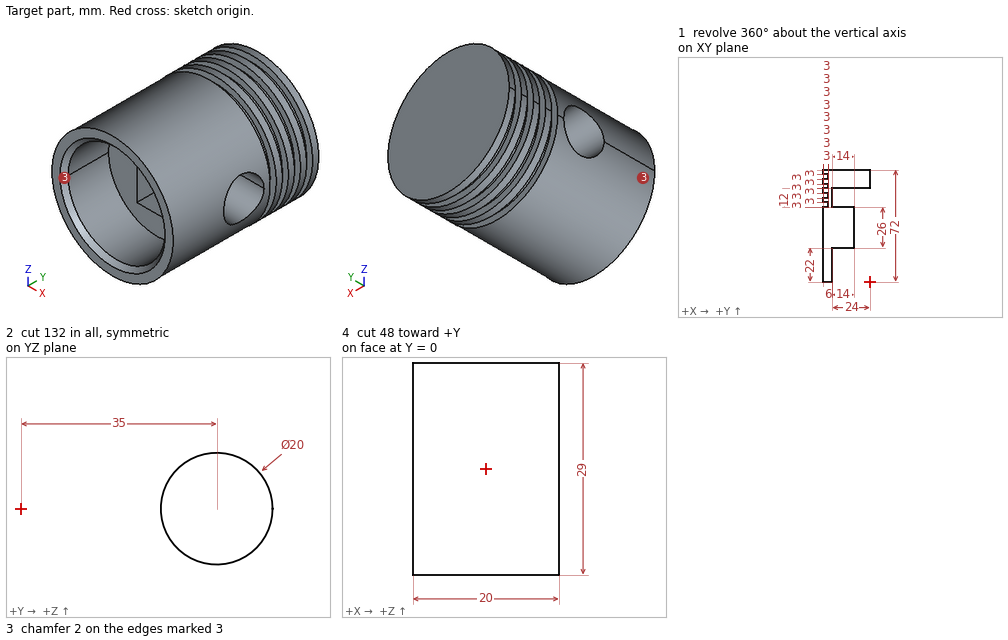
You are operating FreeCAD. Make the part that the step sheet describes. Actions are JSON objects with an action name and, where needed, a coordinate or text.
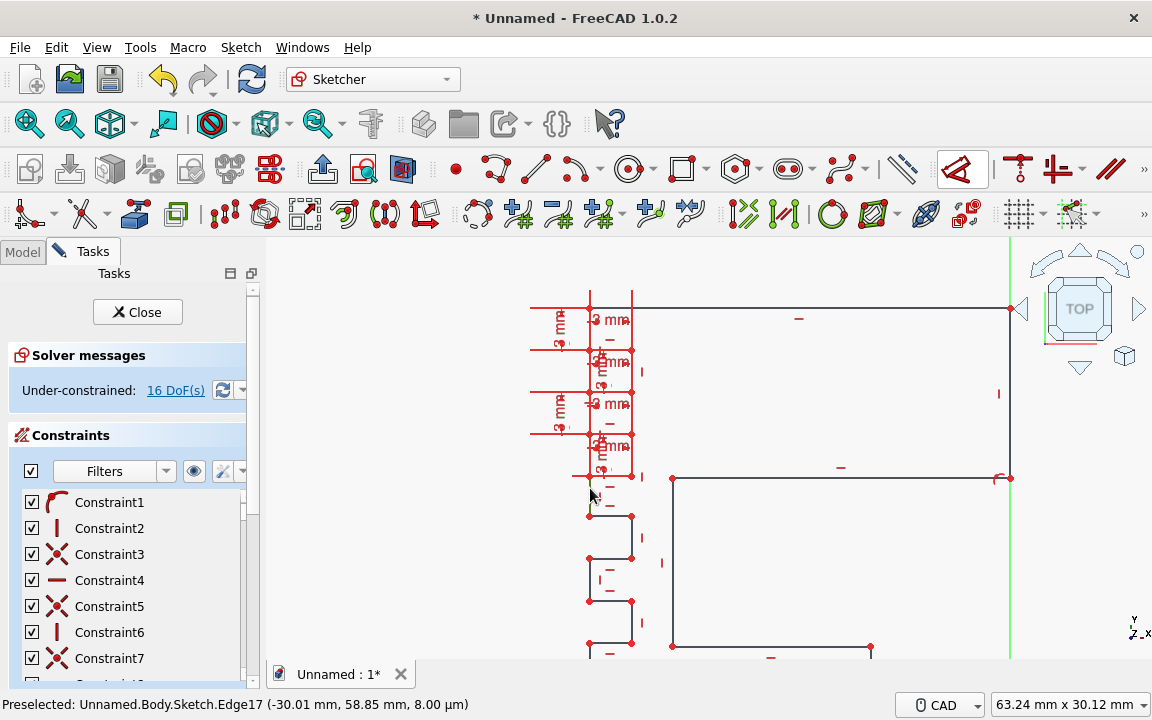
{"action": "key", "text": "i"}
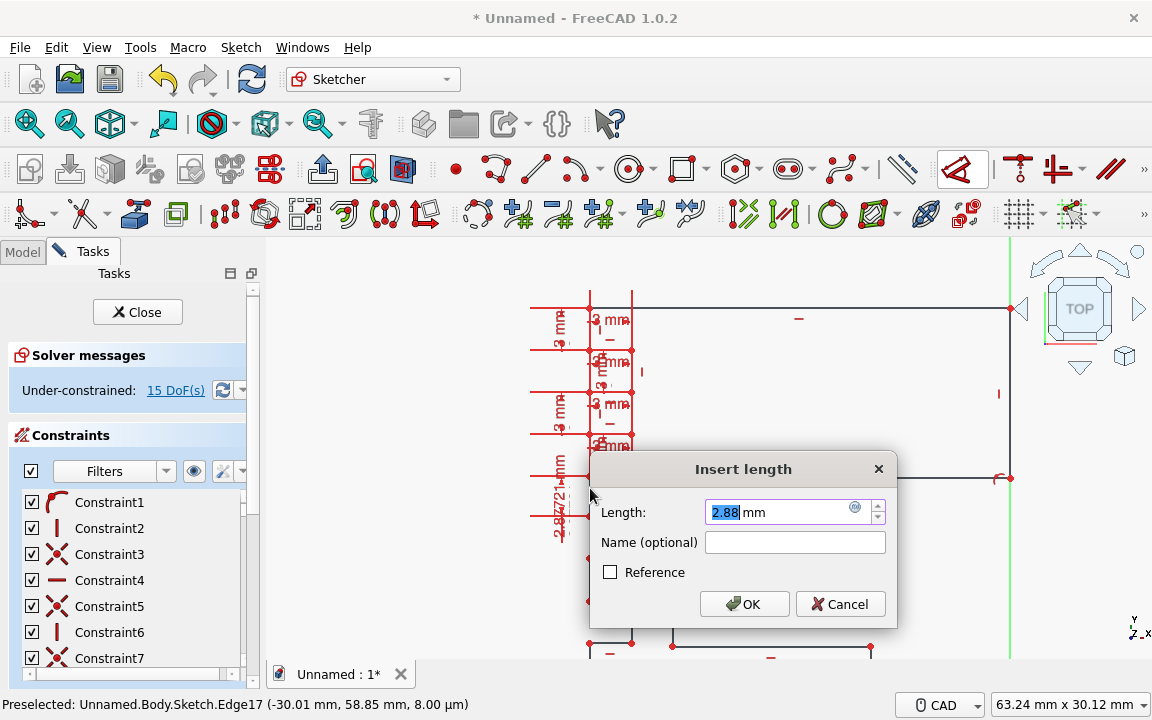
{"action": "type", "text": "3"}
{"action": "key", "text": "Return"}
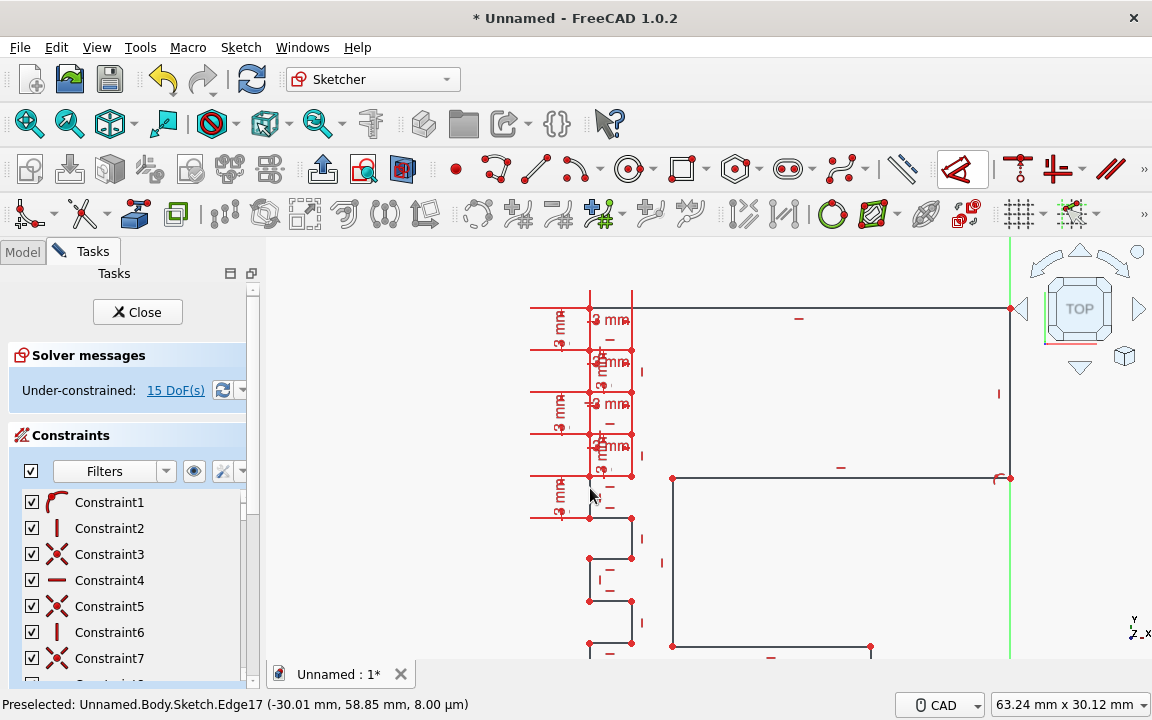
{"action": "left_click", "coordinate": [602, 518]}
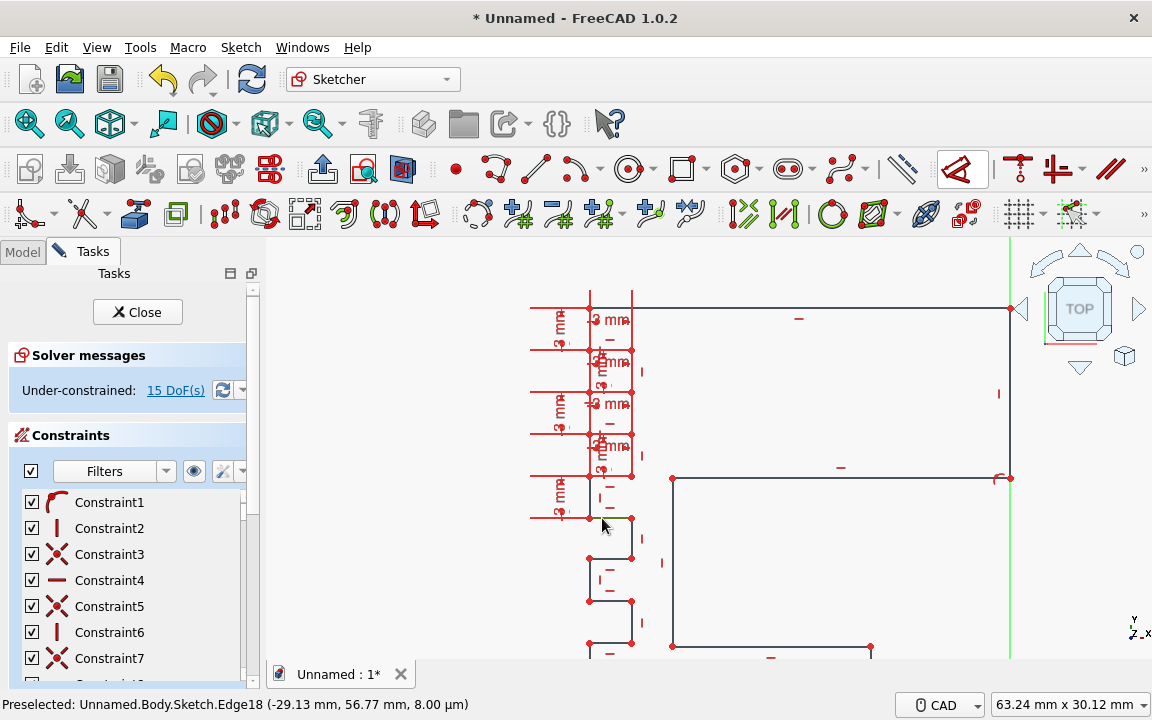
{"action": "key", "text": "l"}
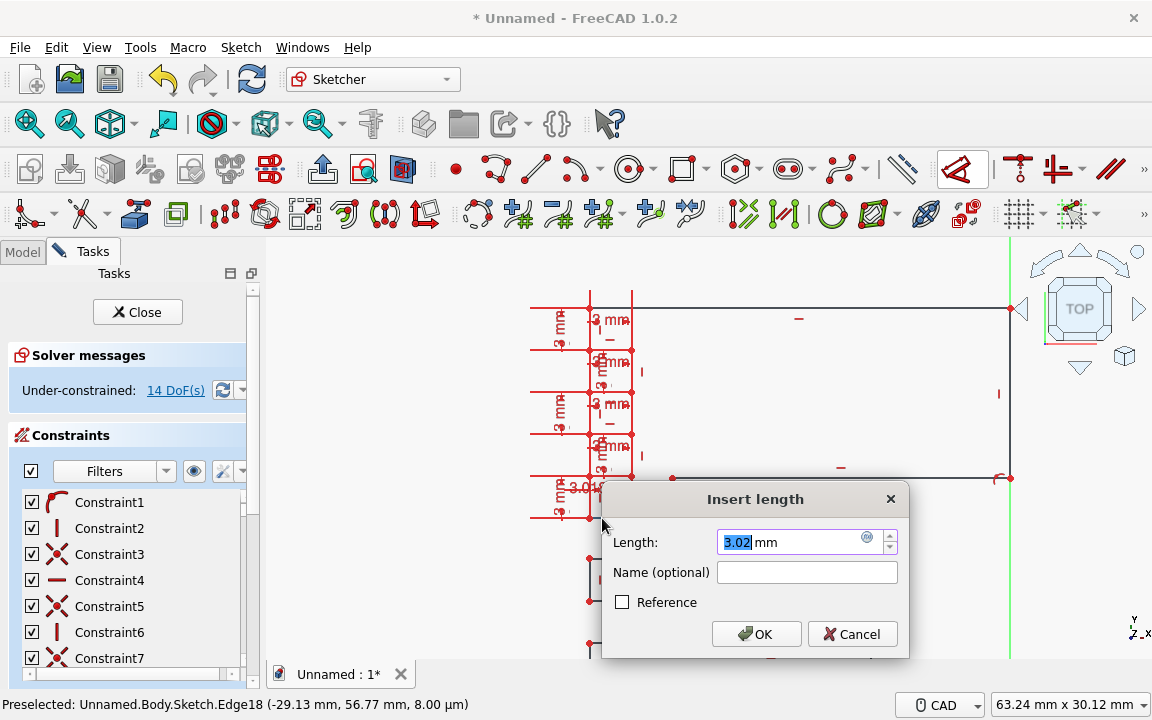
{"action": "type", "text": "3"}
{"action": "key", "text": "Return"}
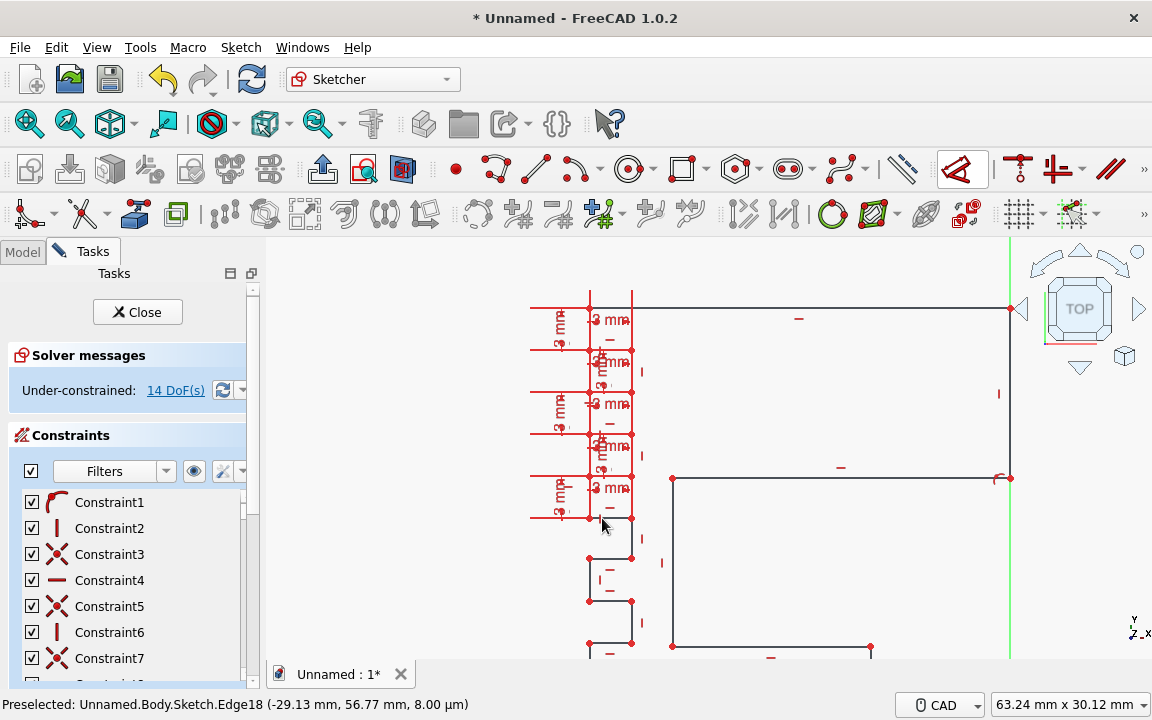
{"action": "left_click", "coordinate": [632, 530]}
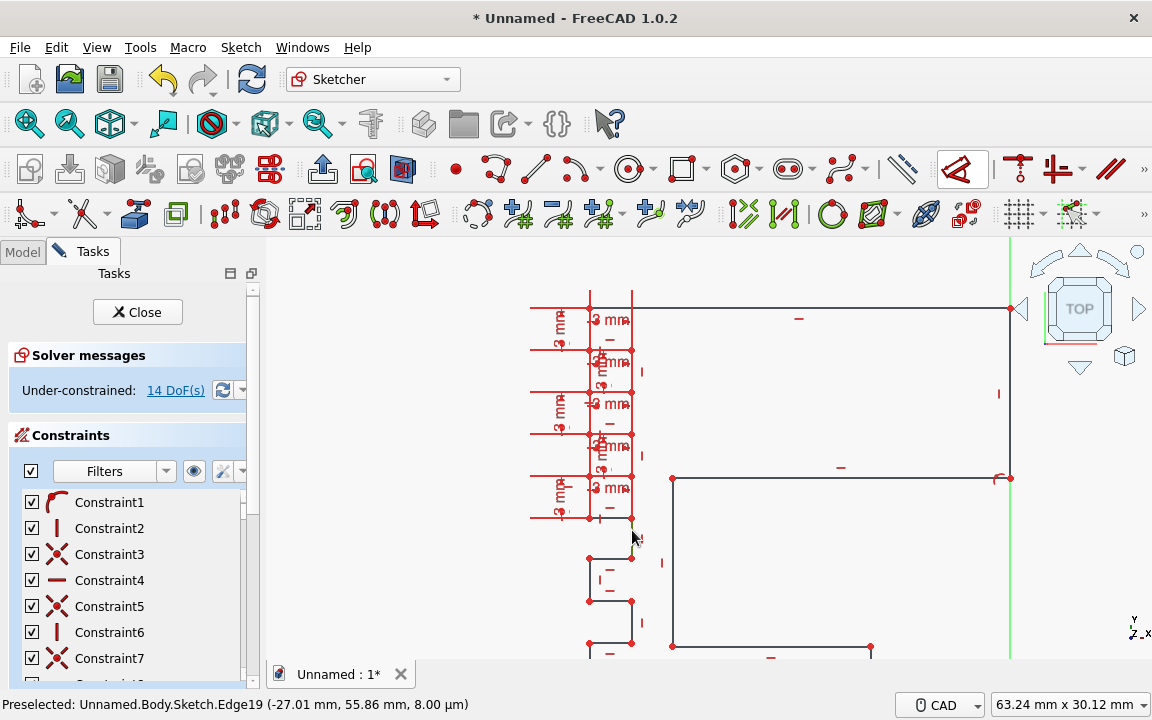
{"action": "key", "text": "i"}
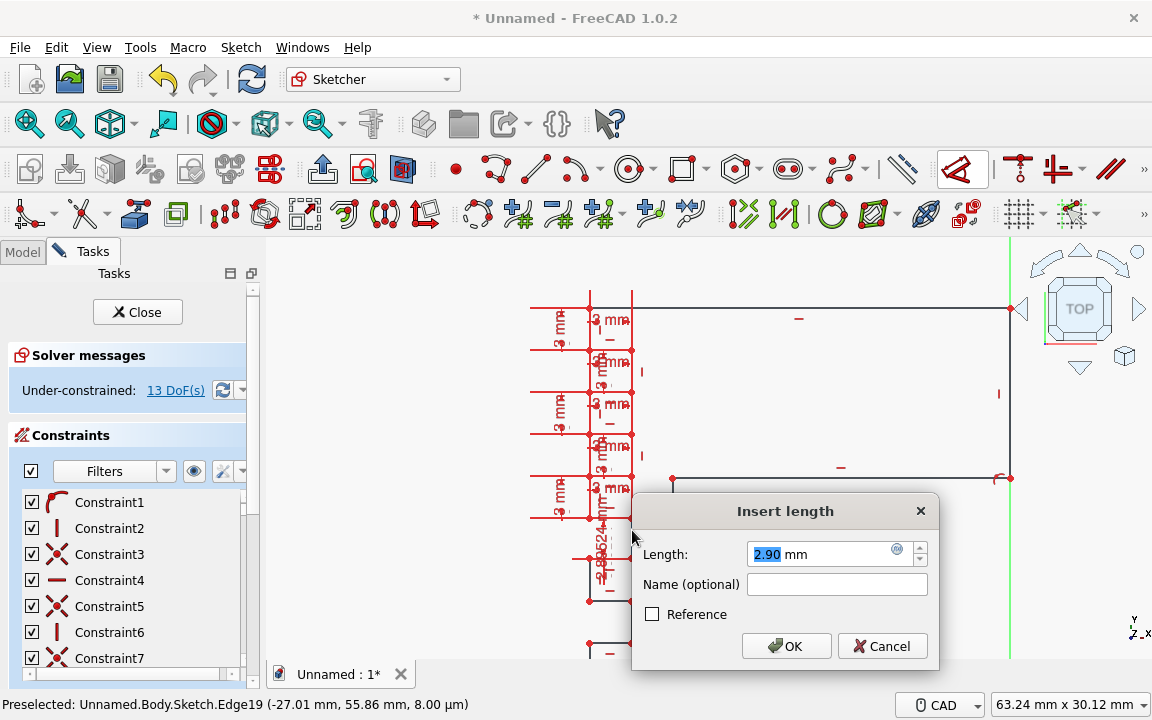
{"action": "type", "text": "3"}
{"action": "key", "text": "Return"}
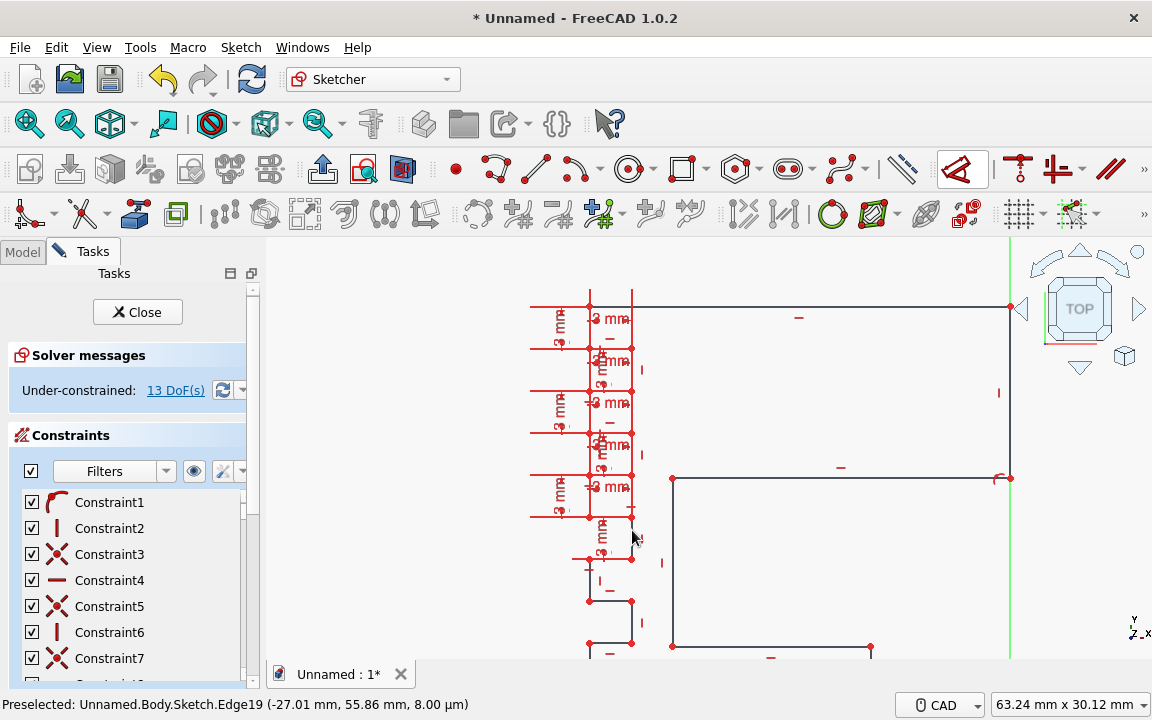
{"action": "left_click", "coordinate": [619, 559]}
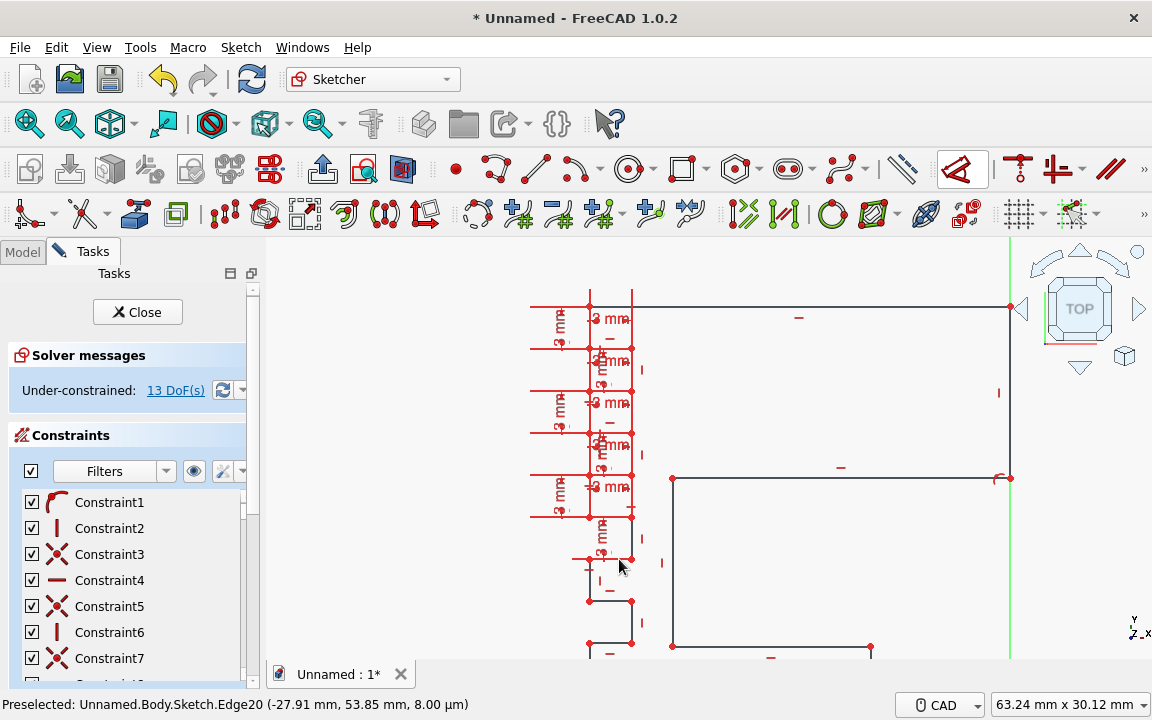
{"action": "key", "text": "l"}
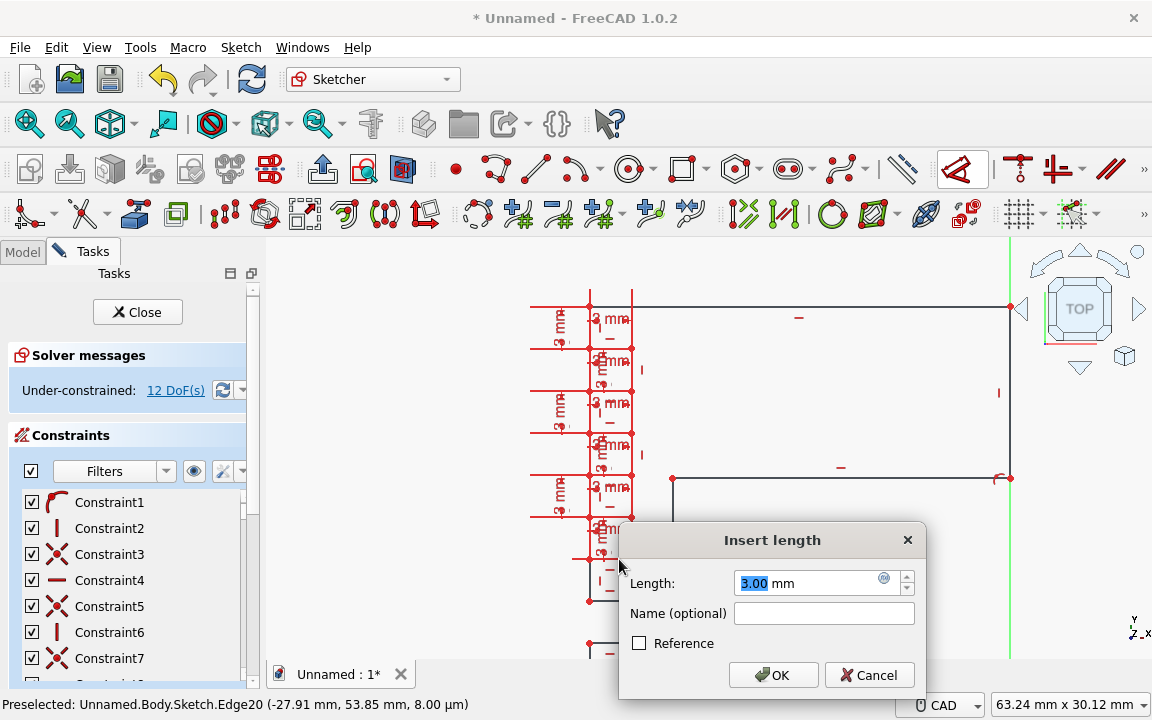
{"action": "type", "text": "3"}
{"action": "key", "text": "Return"}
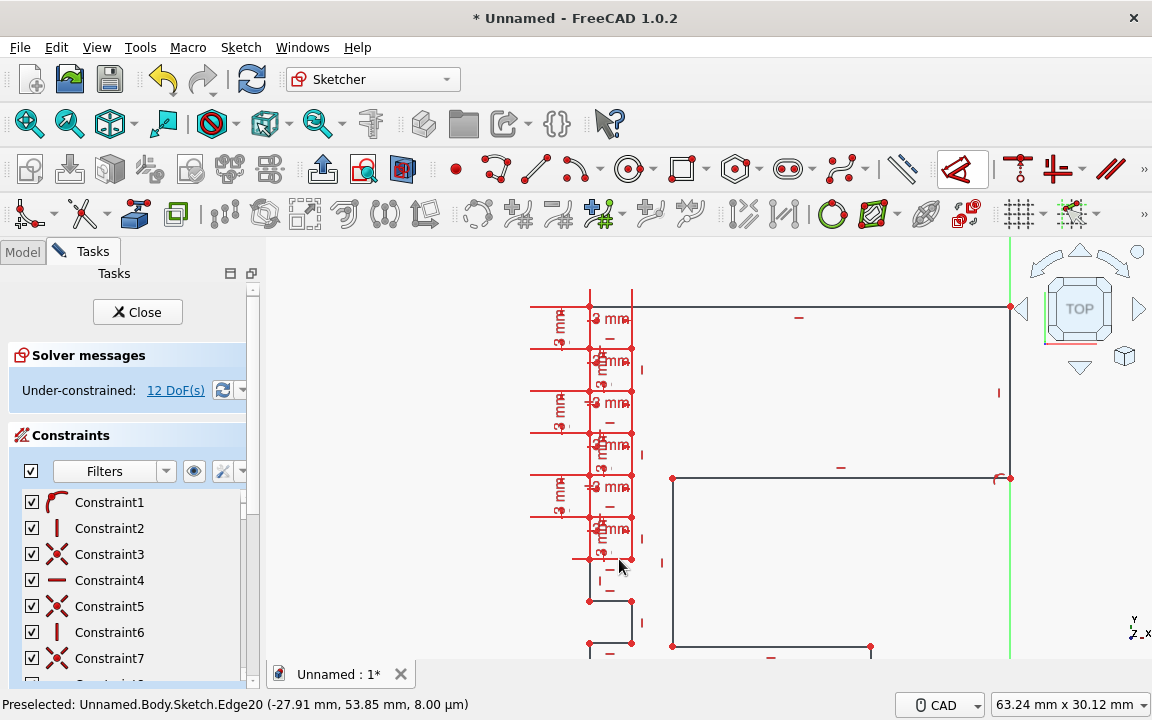
{"action": "left_click", "coordinate": [590, 572]}